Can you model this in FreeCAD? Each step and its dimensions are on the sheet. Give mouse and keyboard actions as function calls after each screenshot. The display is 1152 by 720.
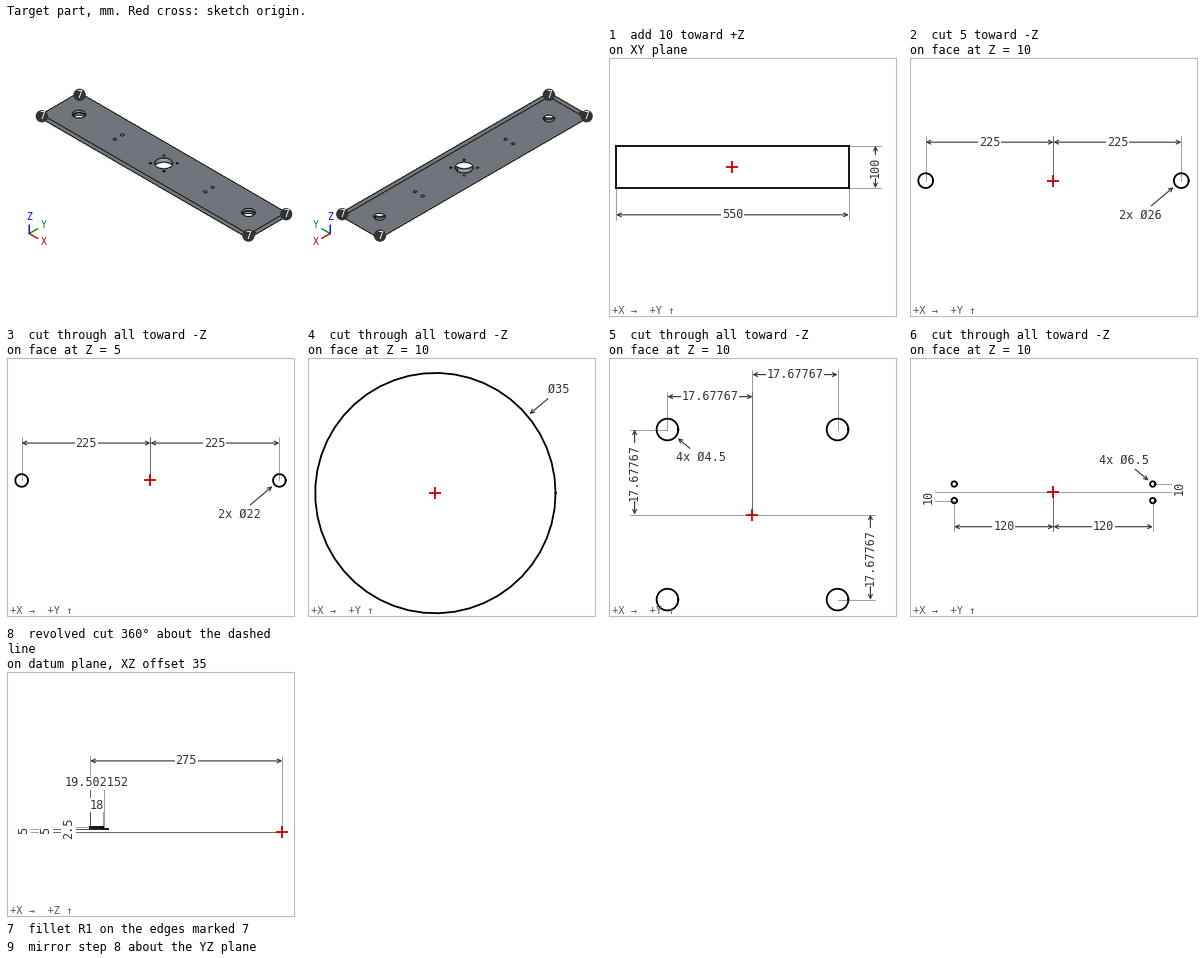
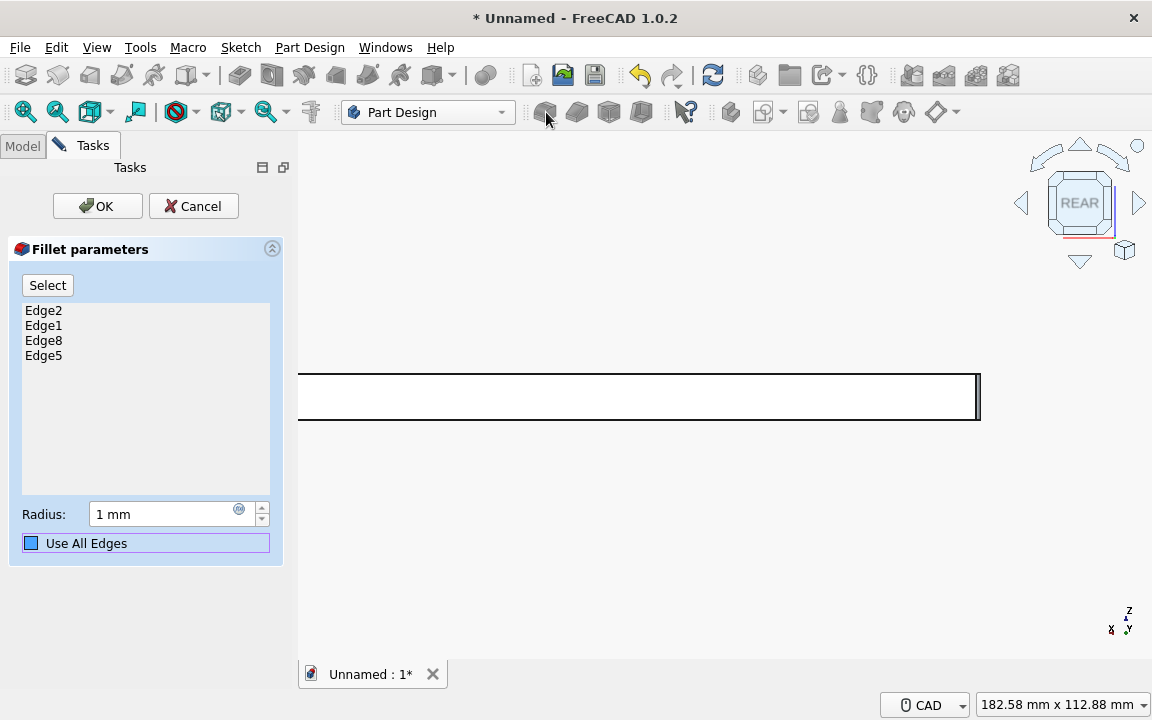
click(98, 206)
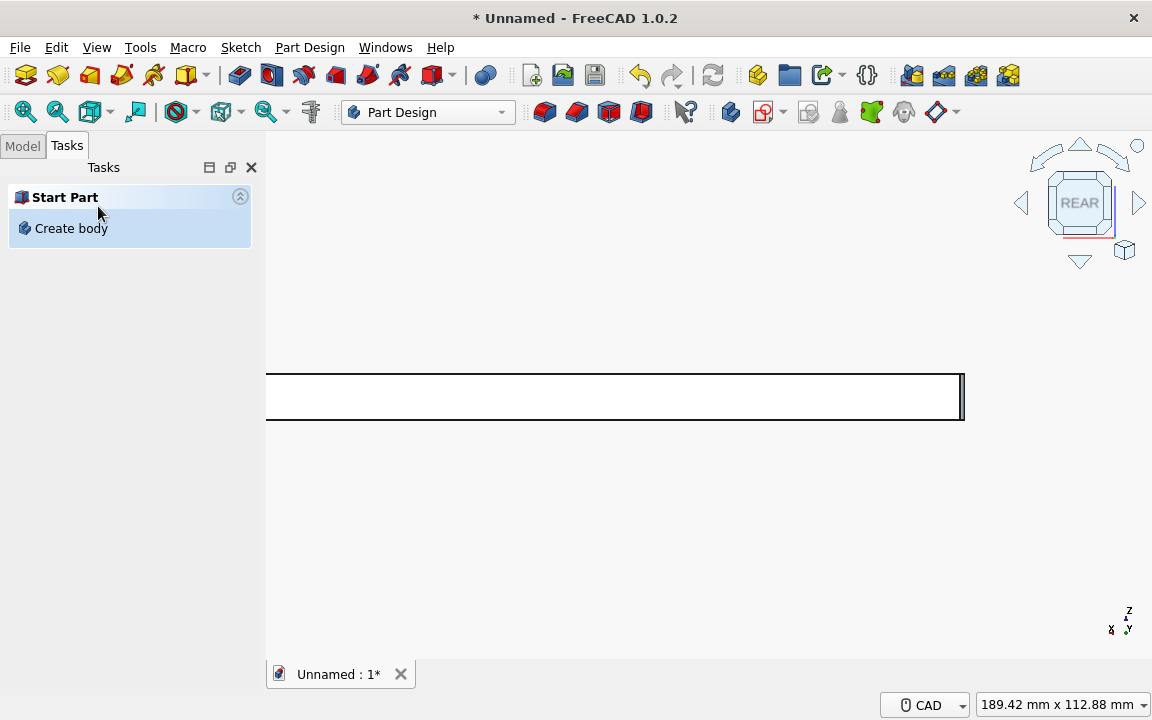
click(26, 112)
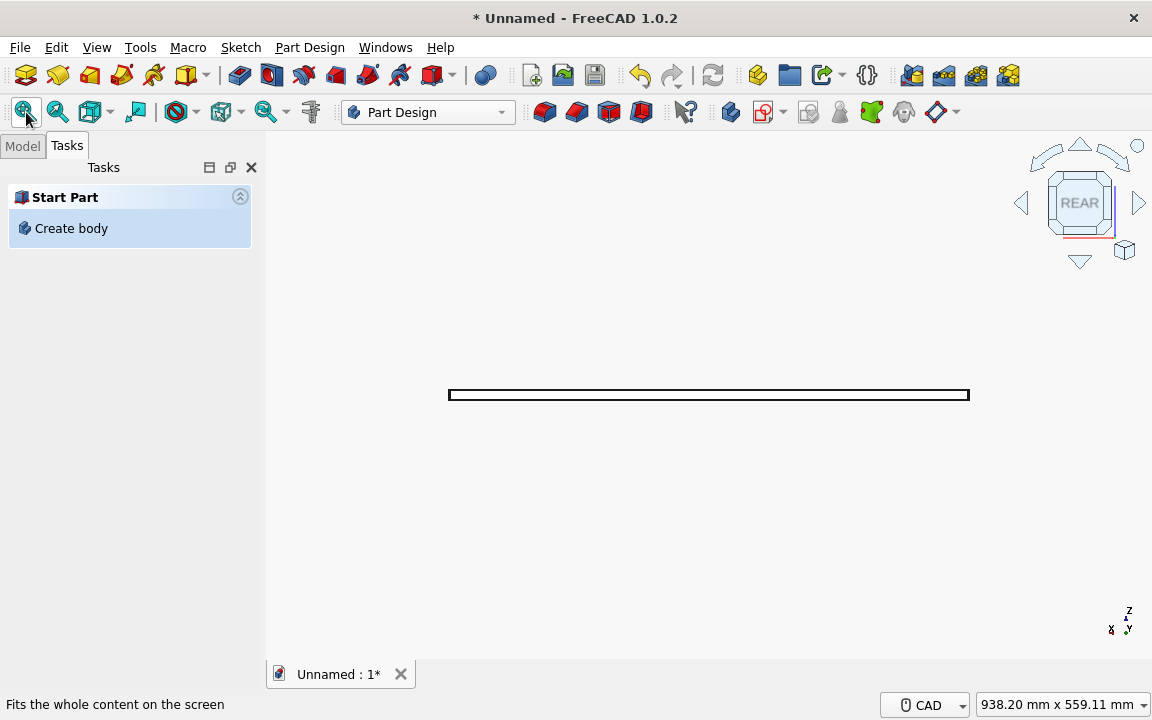
click(23, 145)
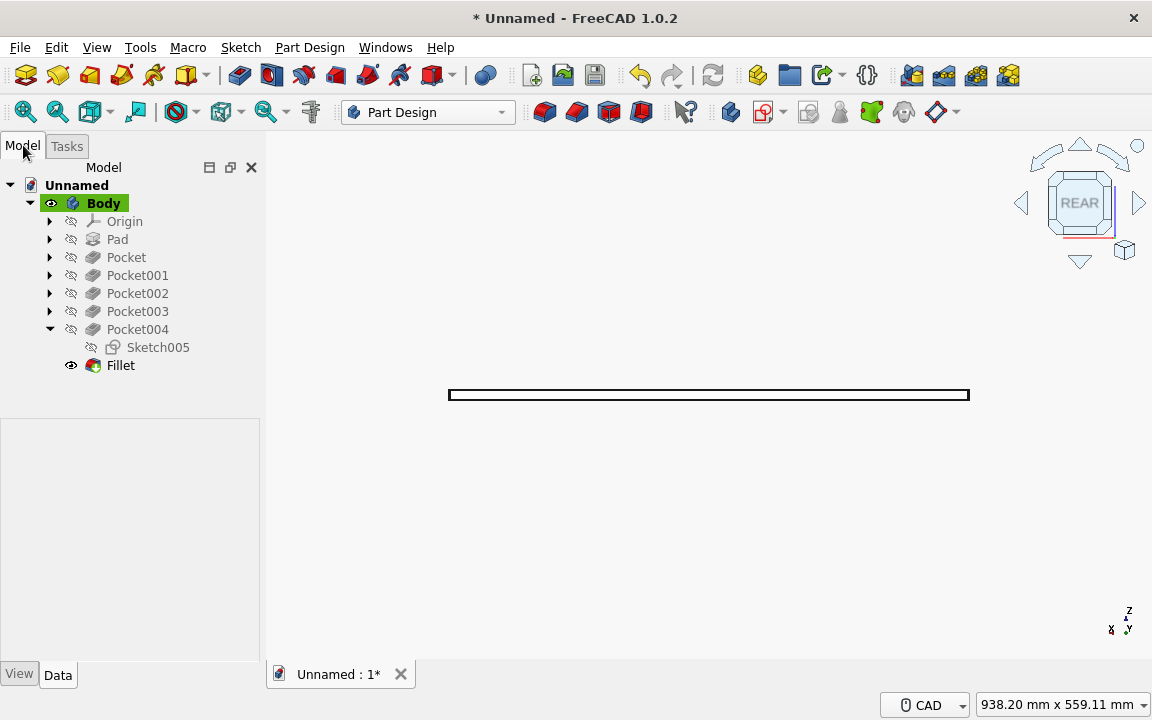
click(50, 221)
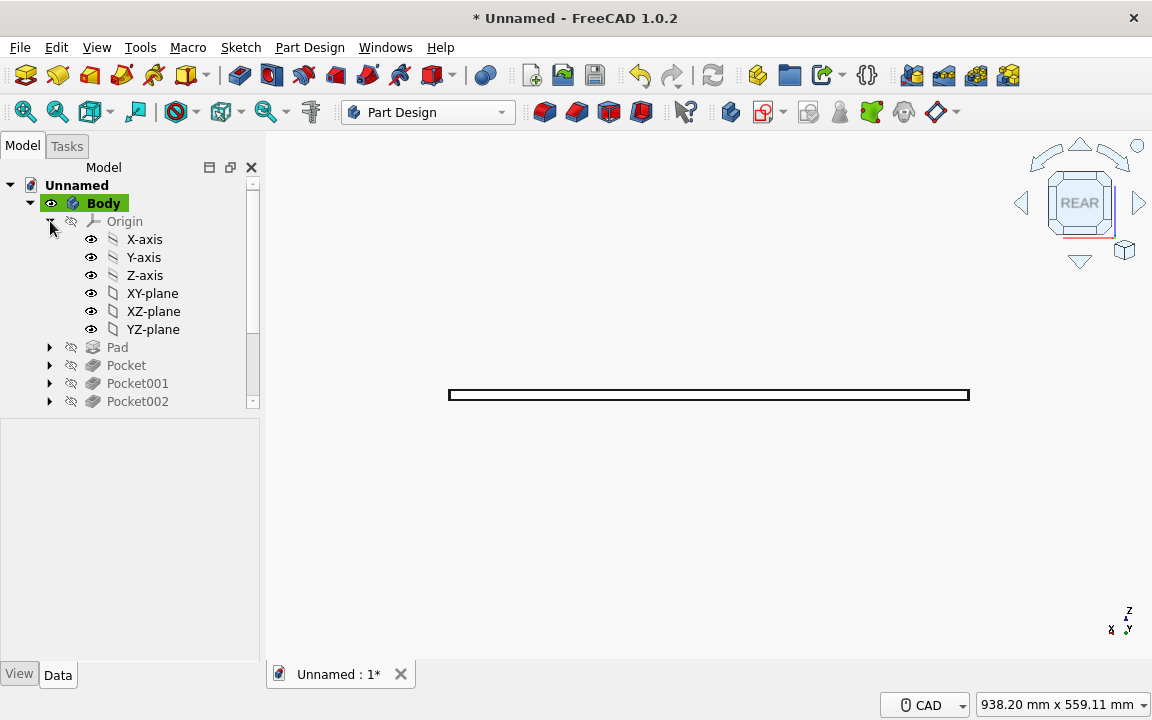
click(136, 311)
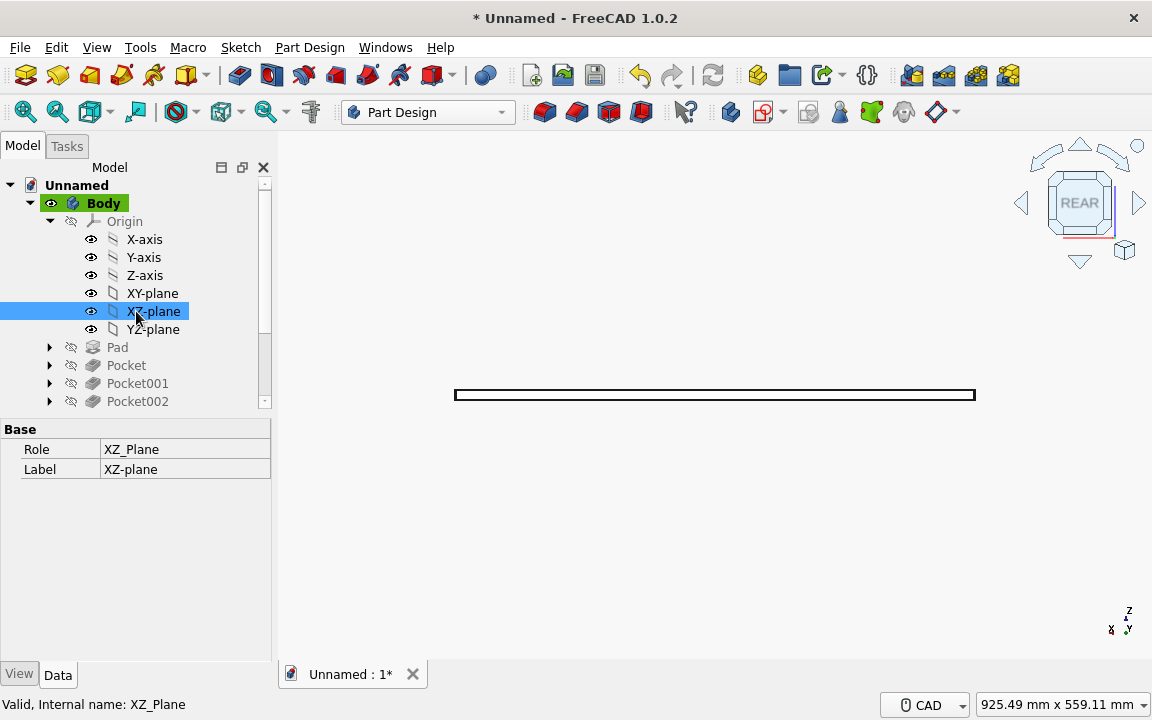
click(936, 112)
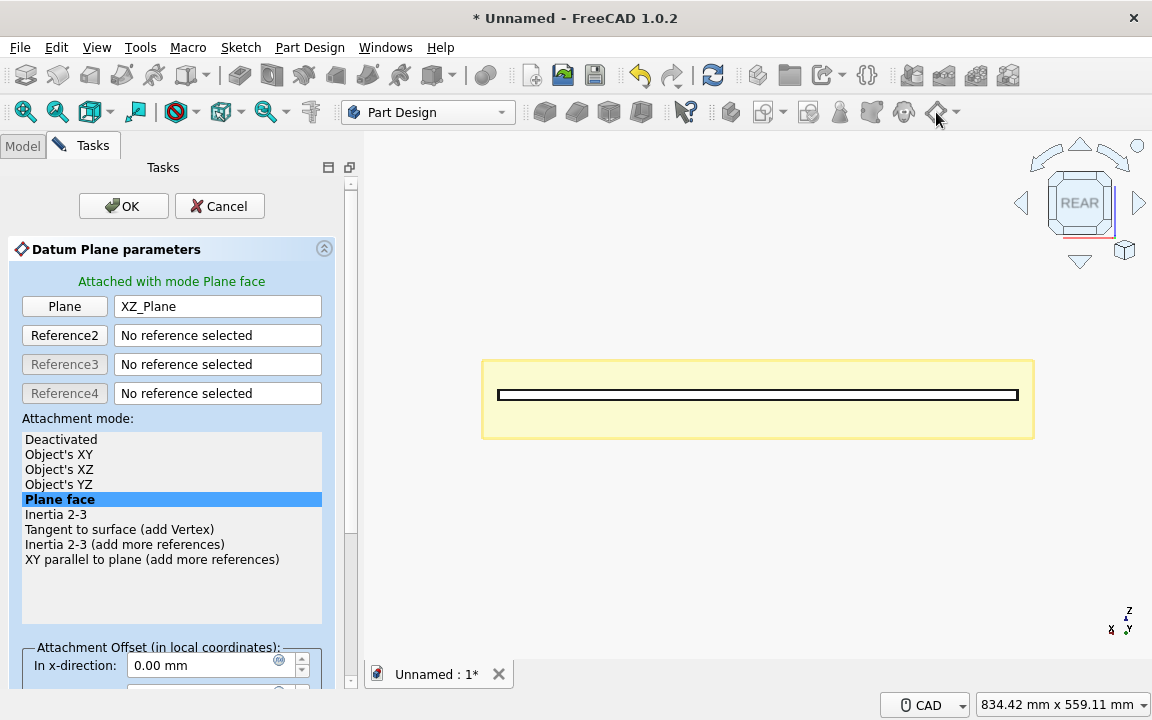
scroll(351, 432, down, 2)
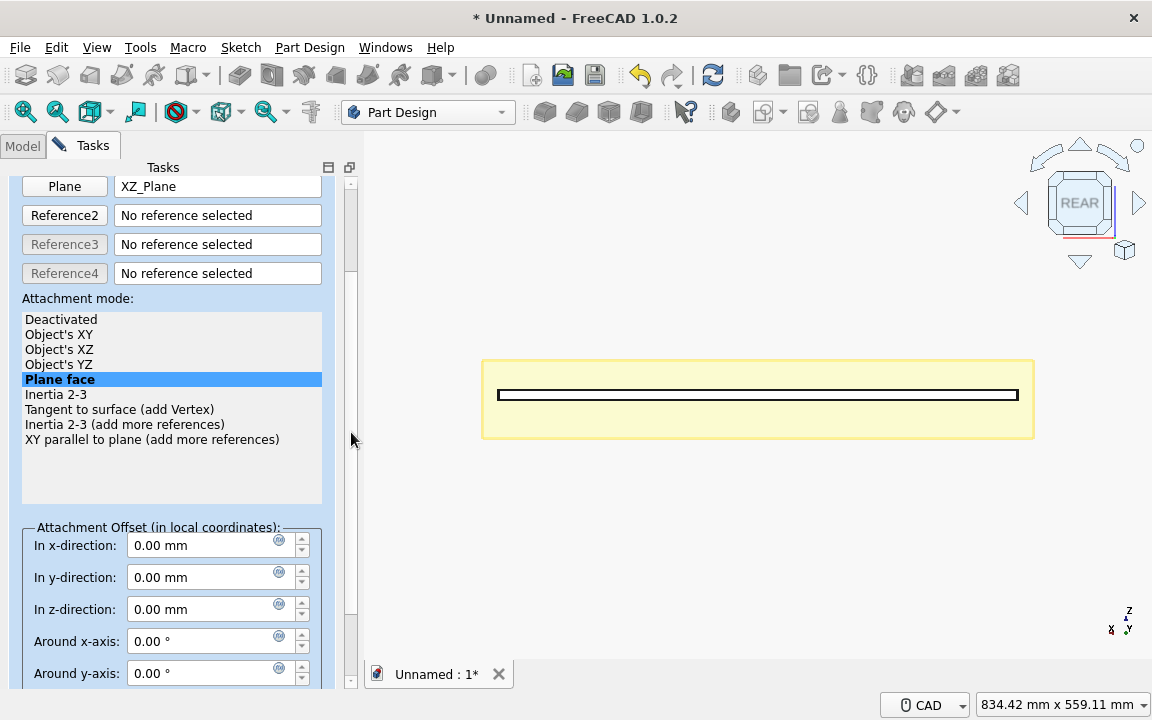
triple_click(210, 609)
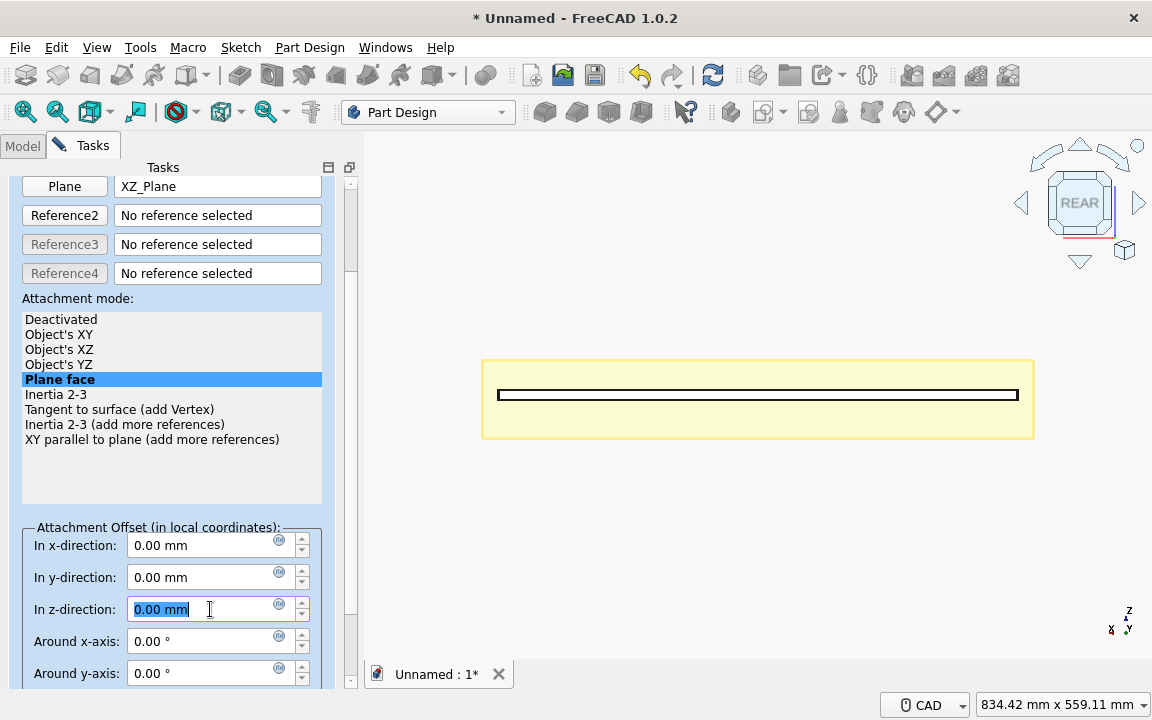
text(35)
key(Tab)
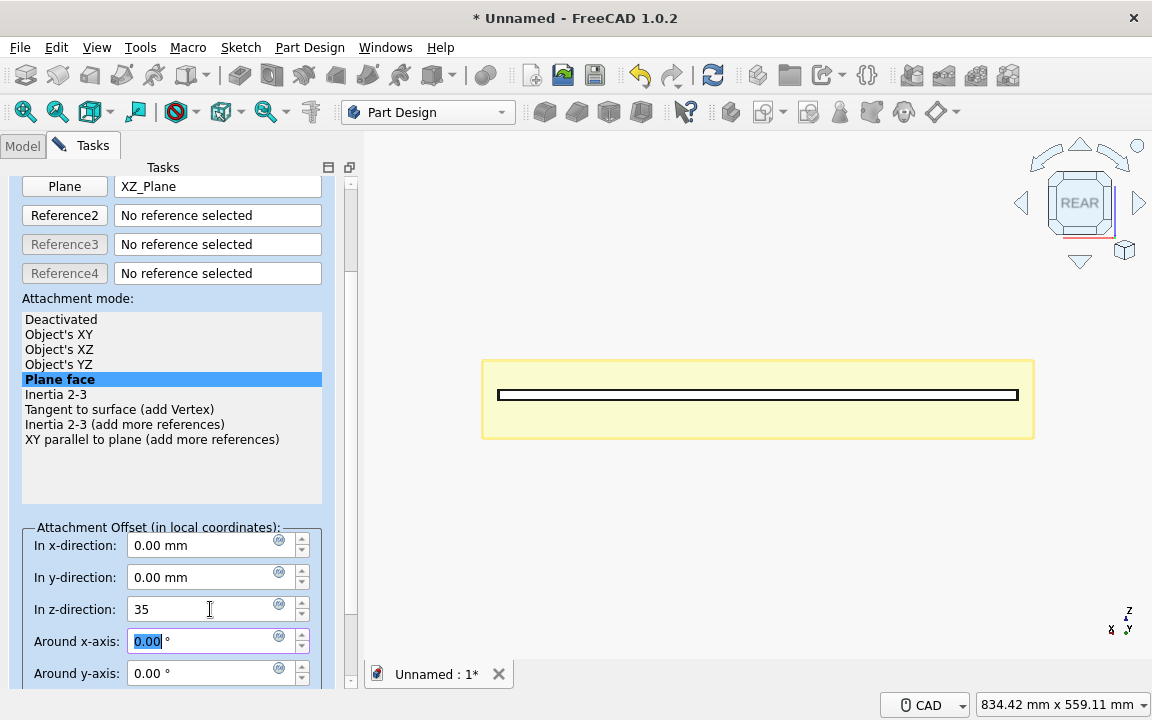
scroll(351, 432, up, 3)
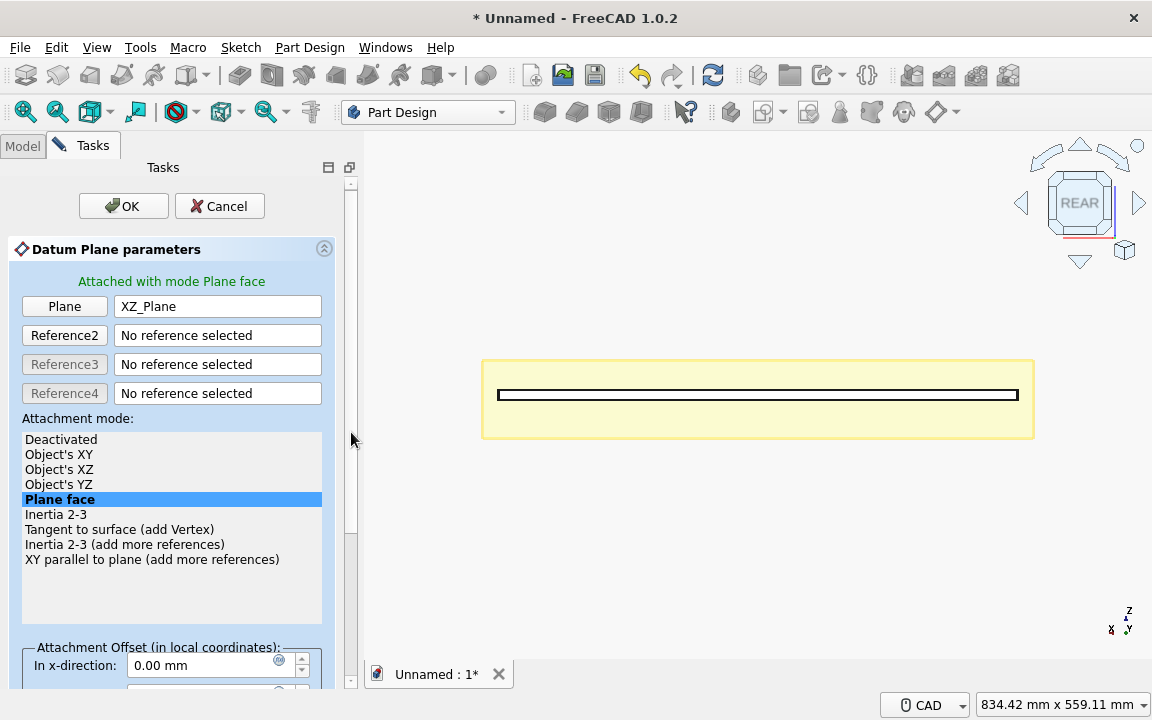
click(124, 206)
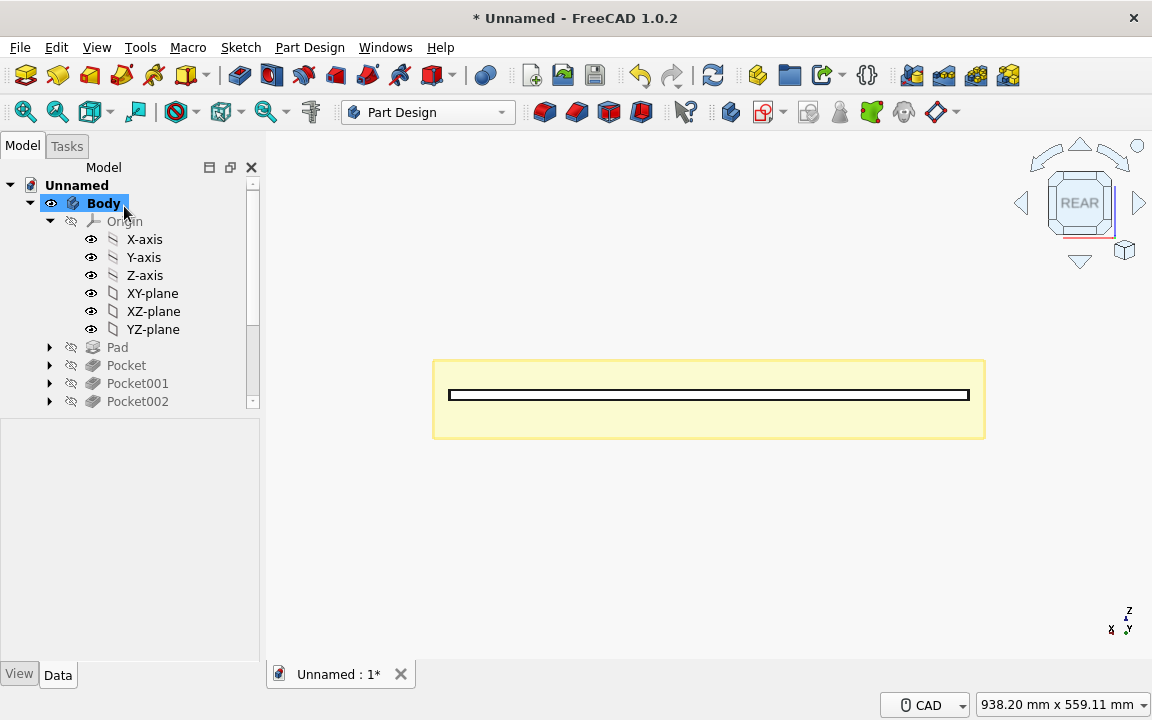
scroll(100, 289, down, 3)